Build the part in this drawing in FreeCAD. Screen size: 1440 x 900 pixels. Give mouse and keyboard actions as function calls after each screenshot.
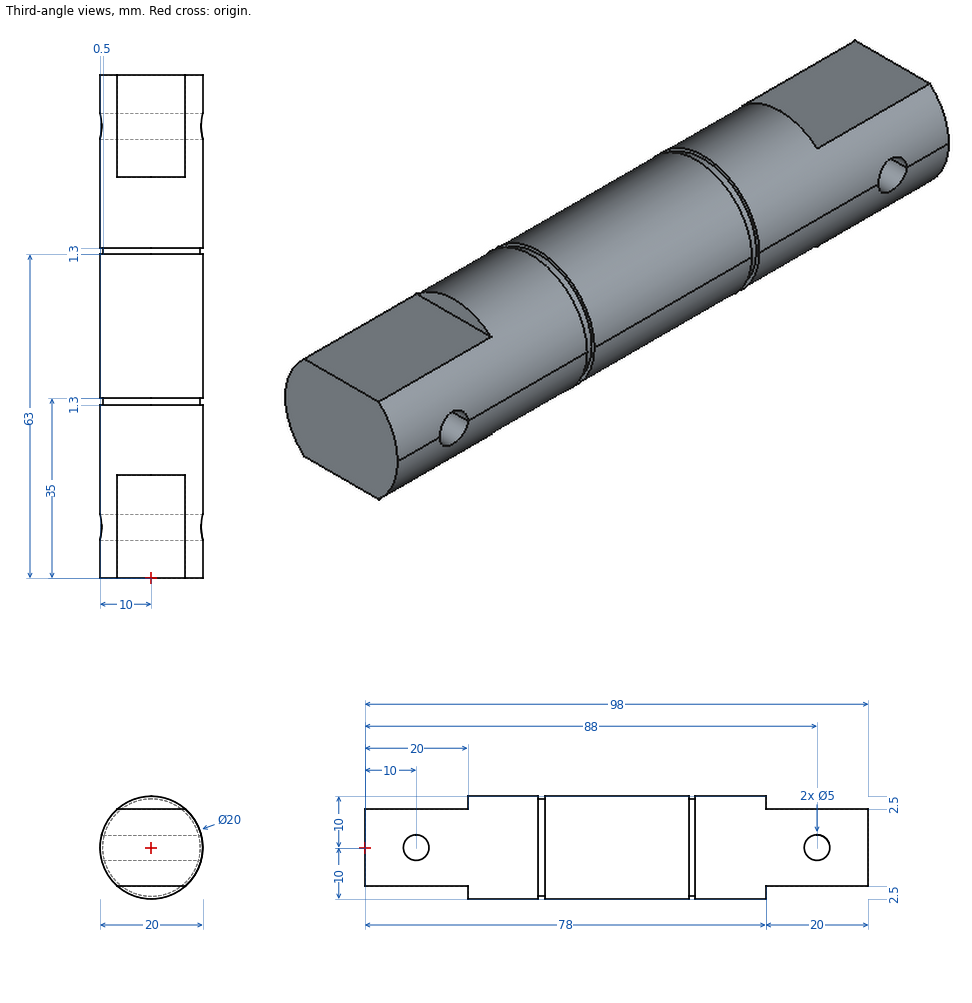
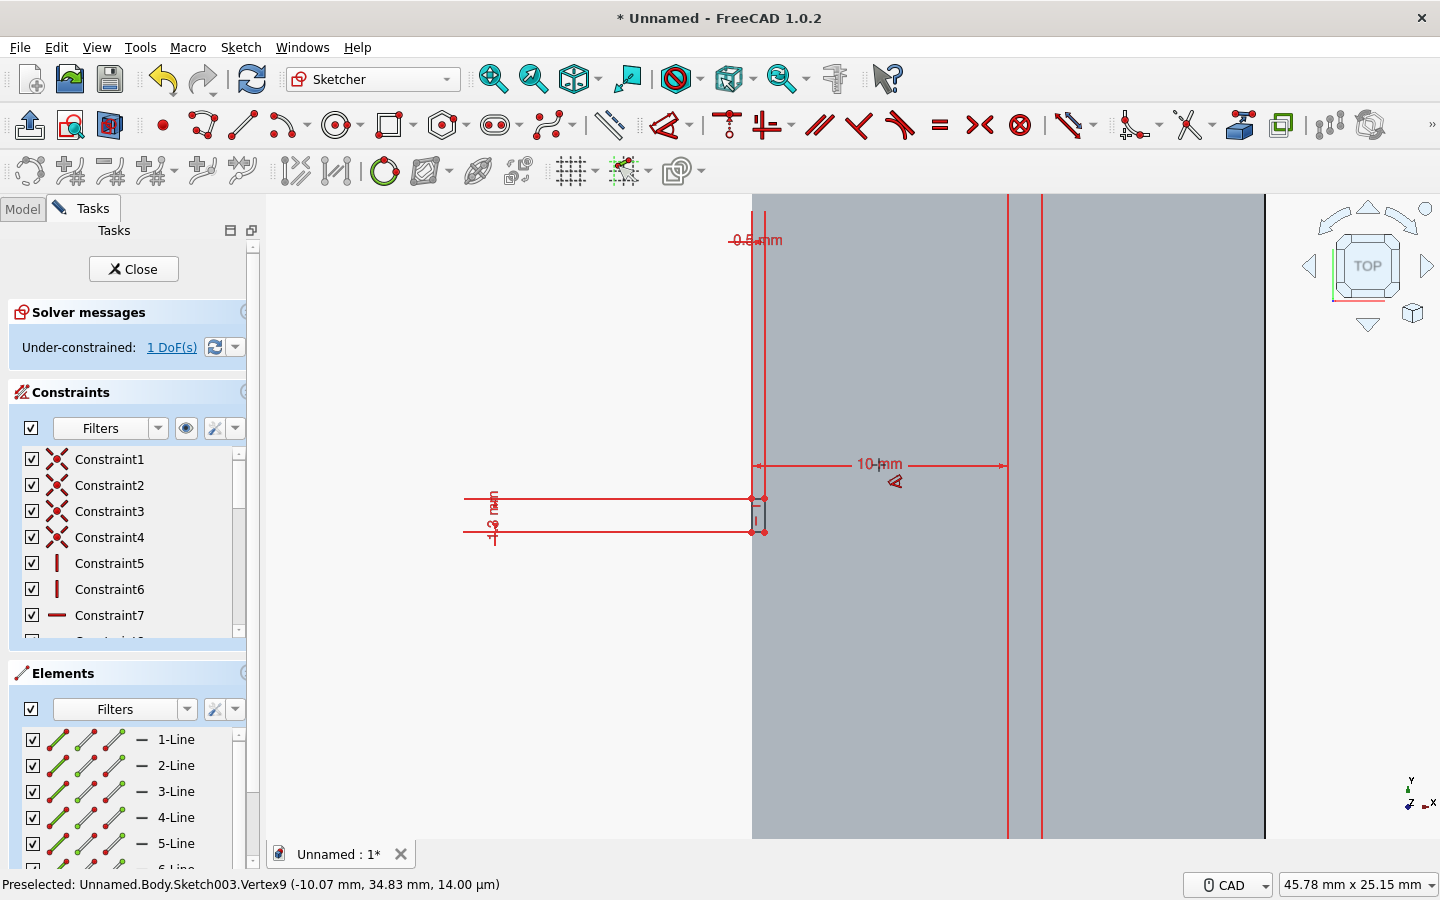
click(752, 499)
click(1042, 655)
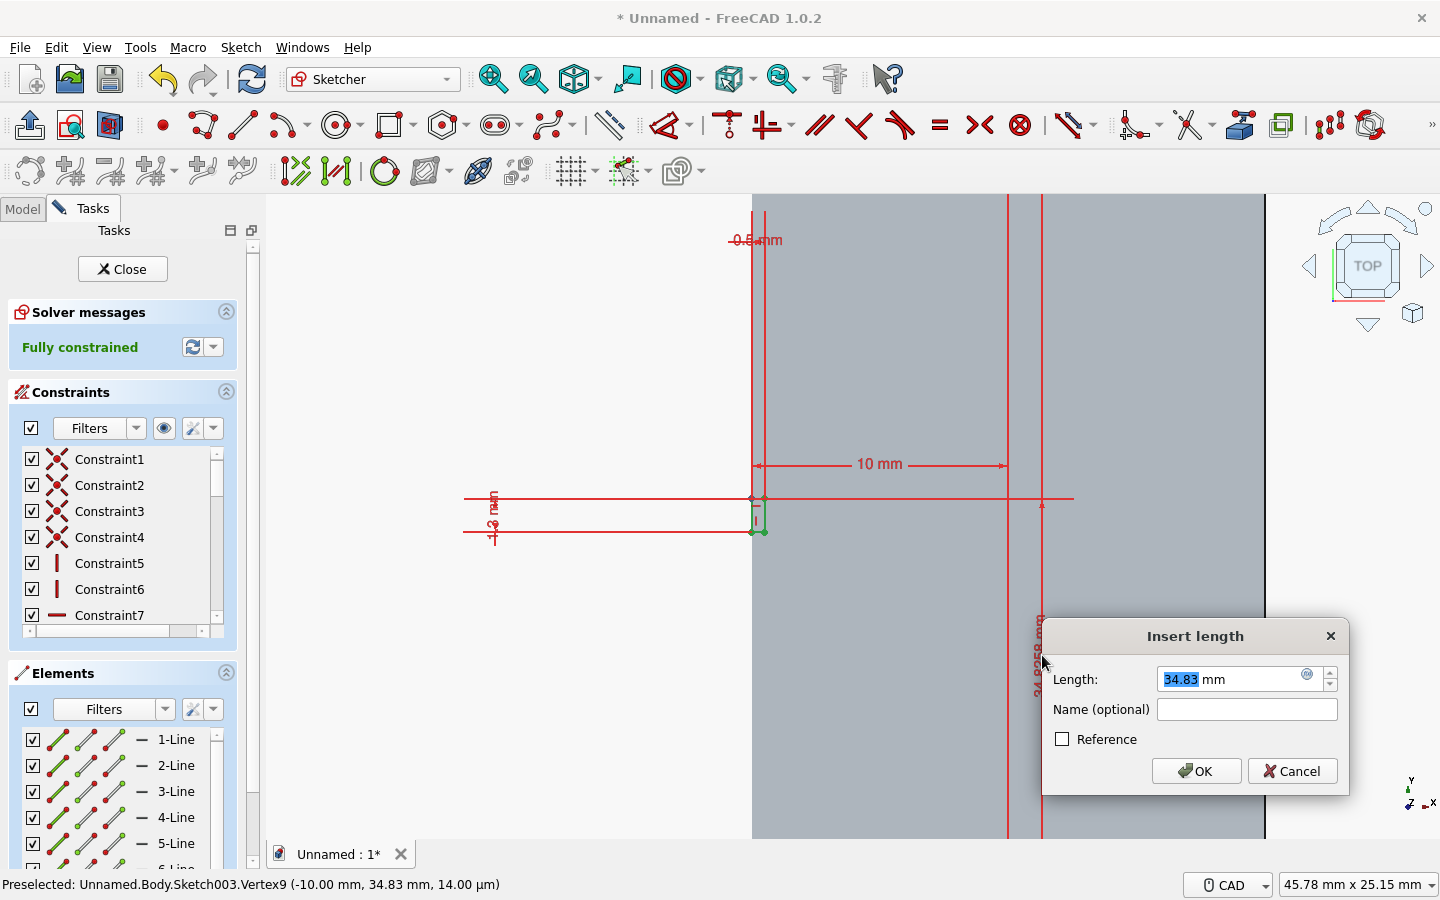
text(35)
key(Return)
key(Escape)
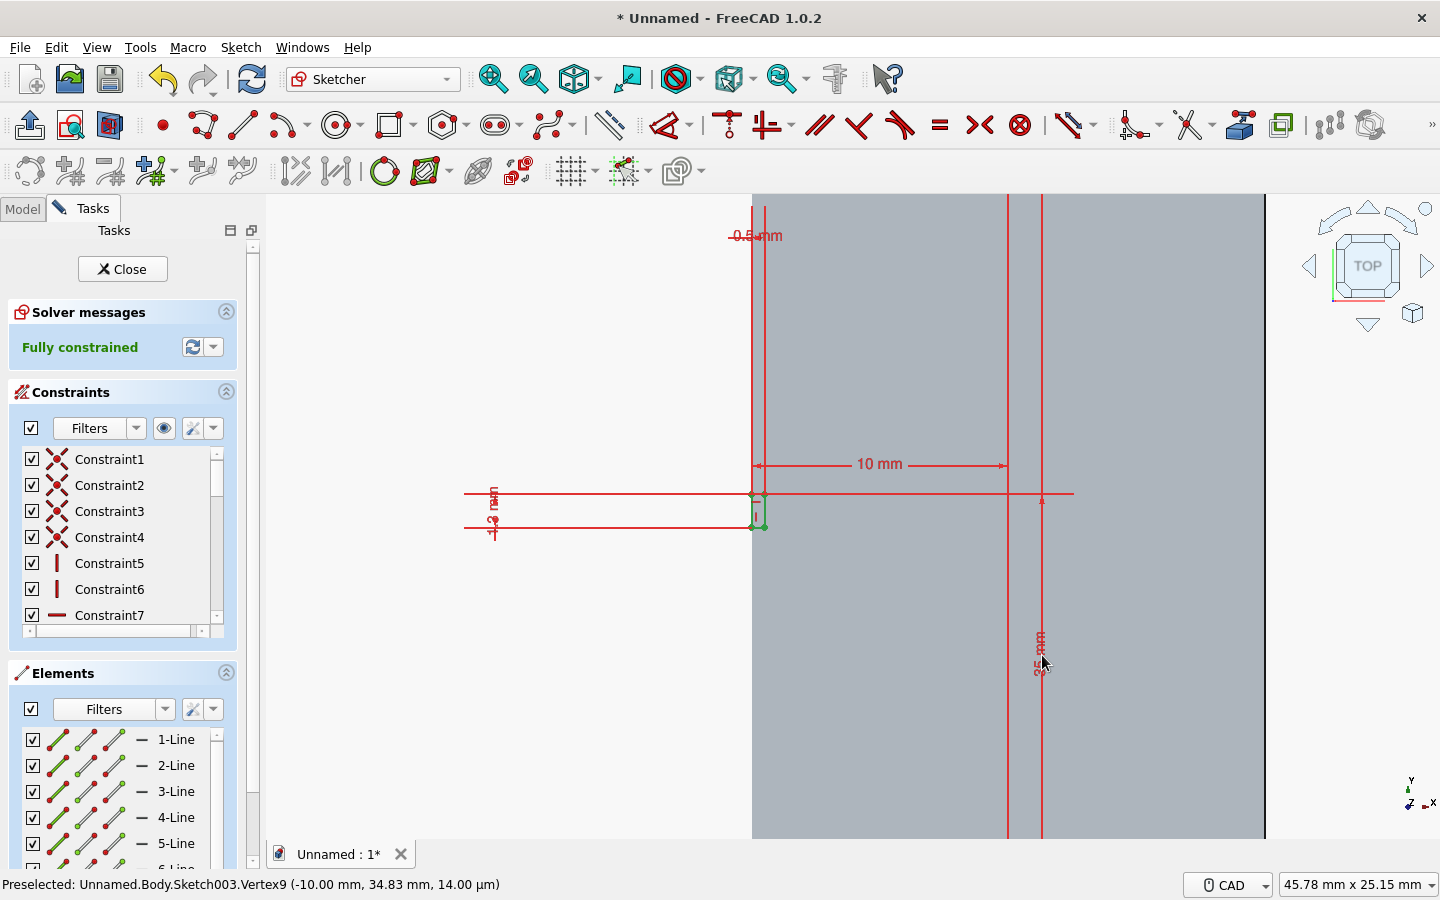
click(123, 269)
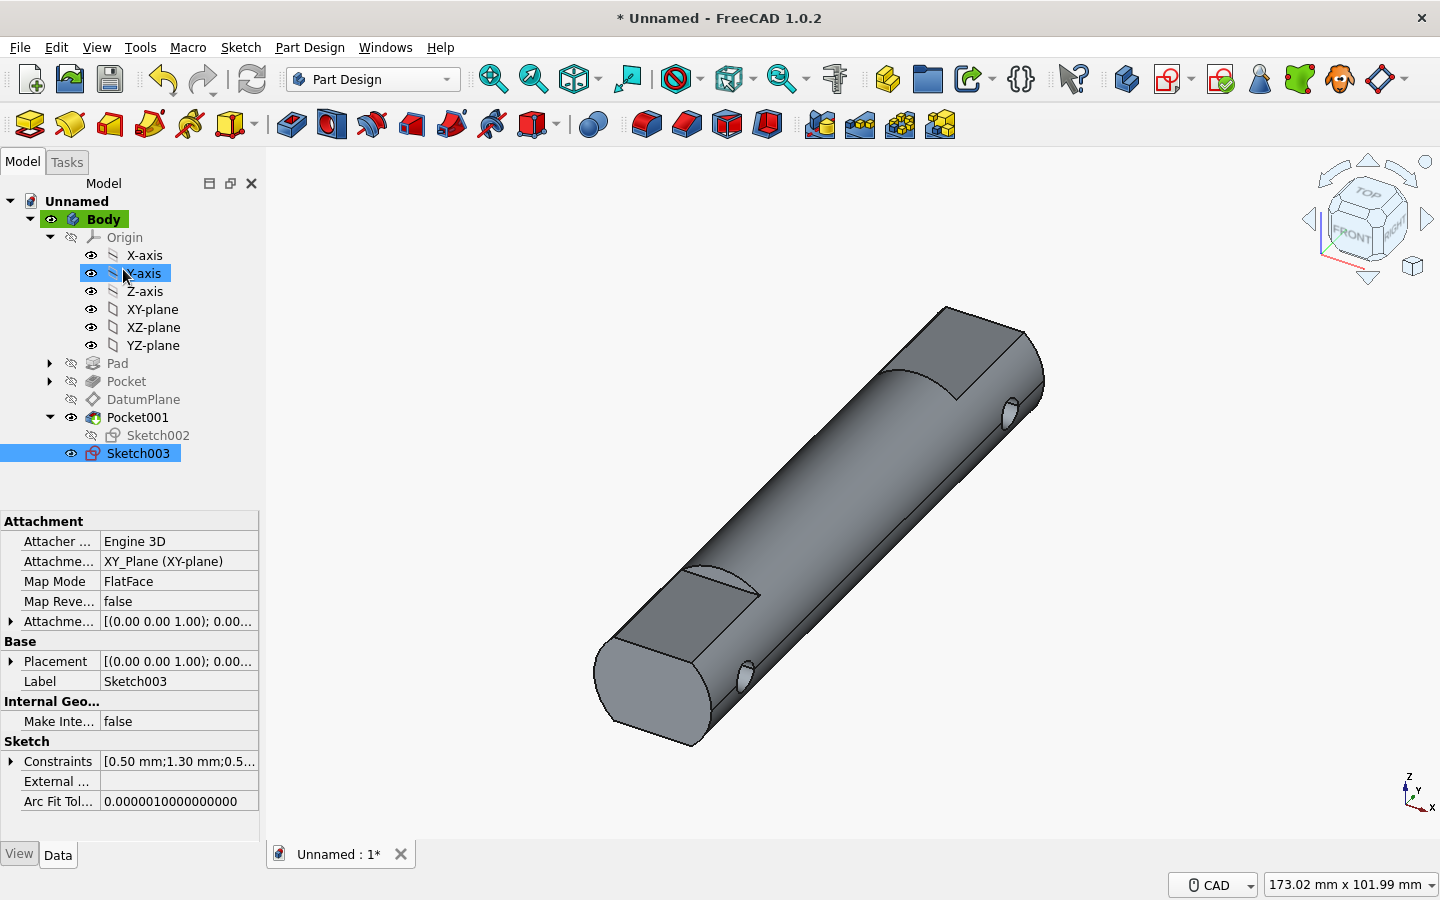
click(372, 124)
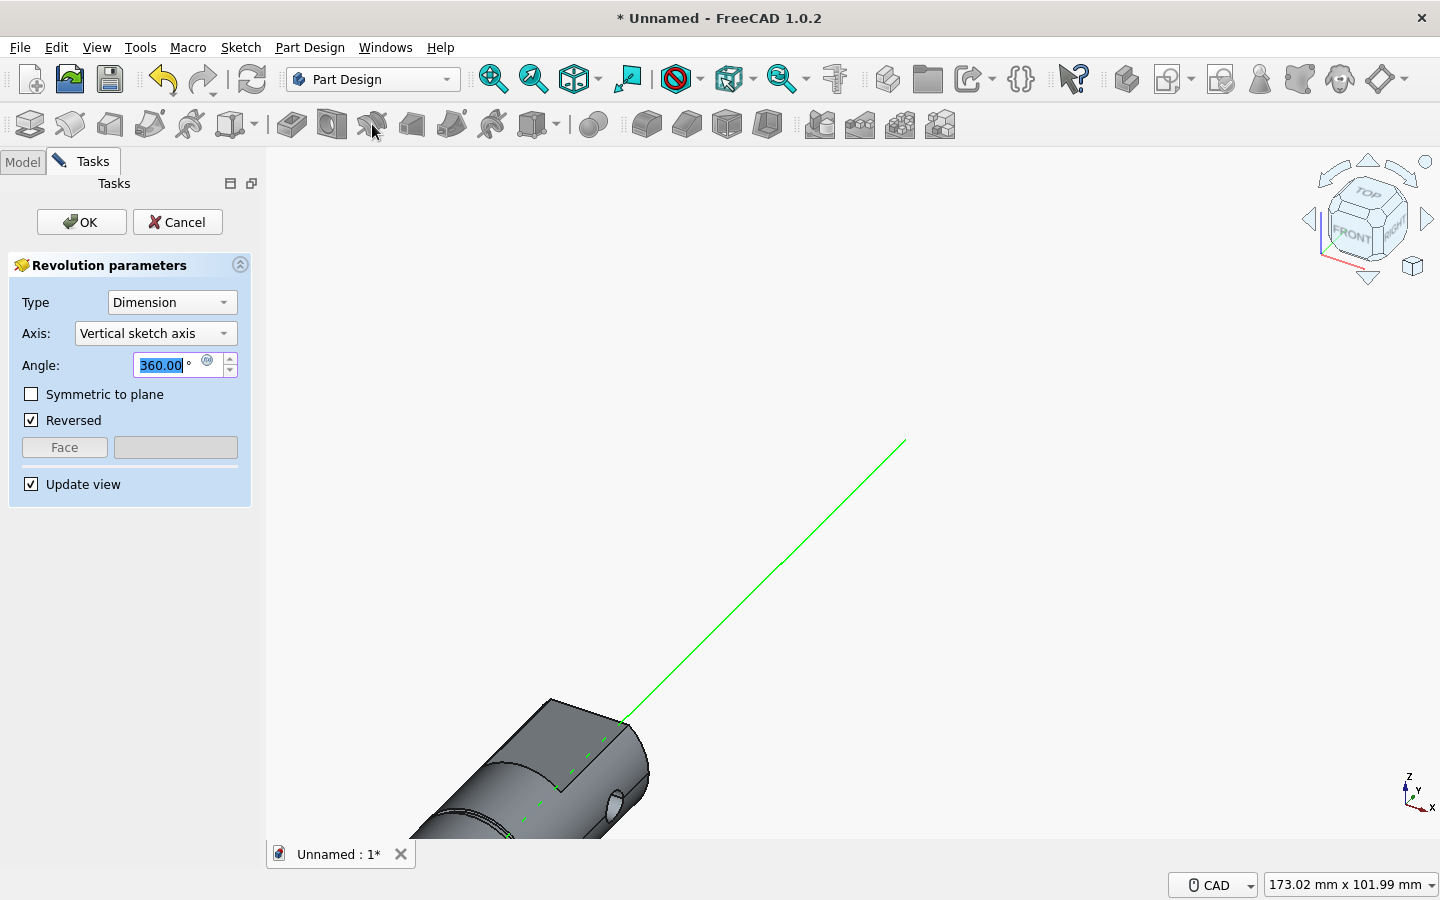
click(82, 222)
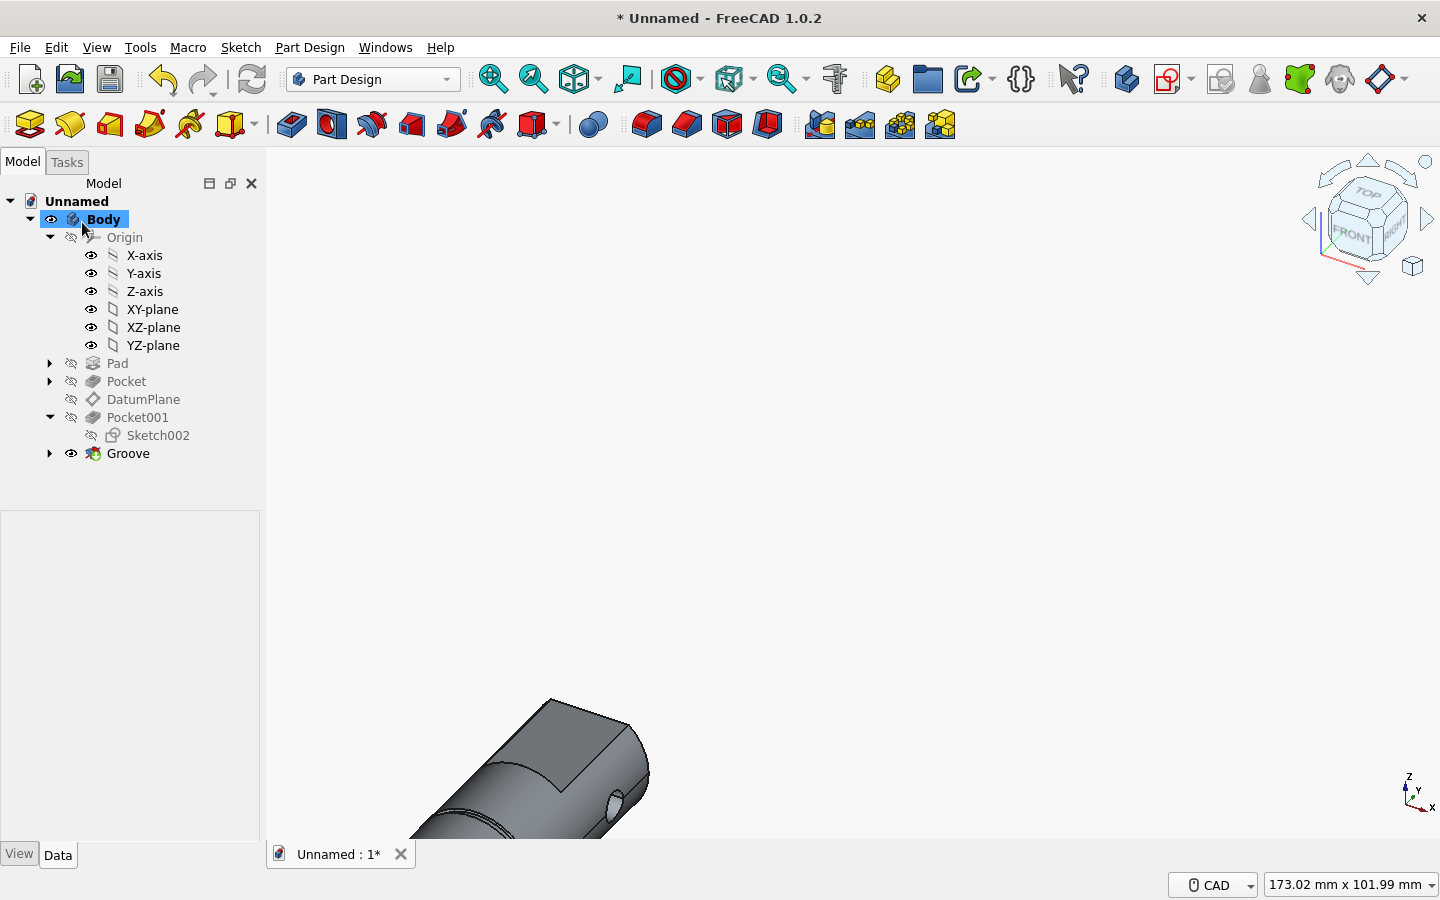
key(0)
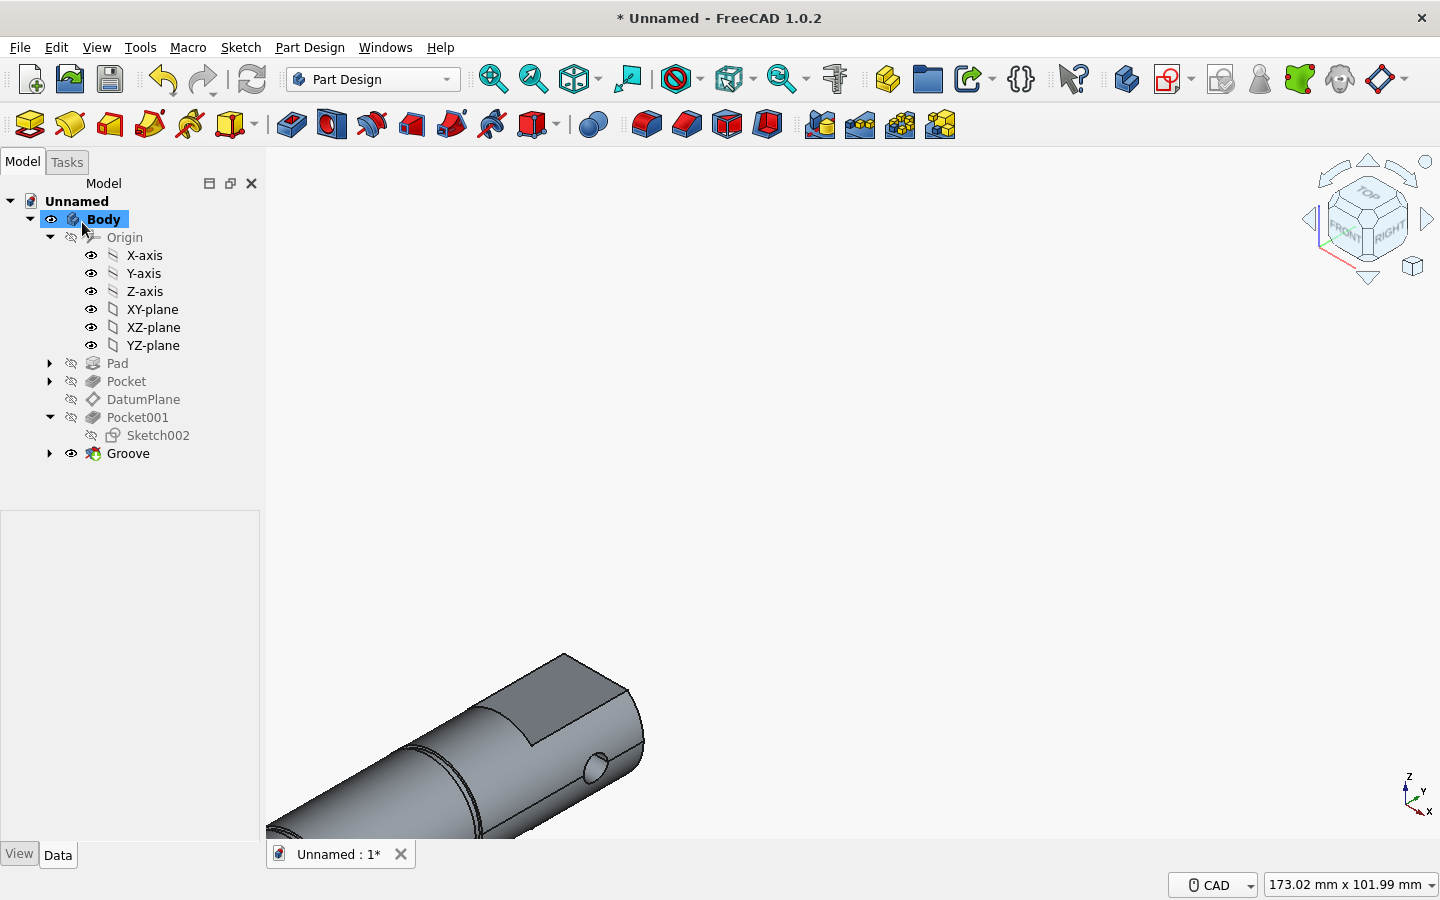
key(v)
key(f)